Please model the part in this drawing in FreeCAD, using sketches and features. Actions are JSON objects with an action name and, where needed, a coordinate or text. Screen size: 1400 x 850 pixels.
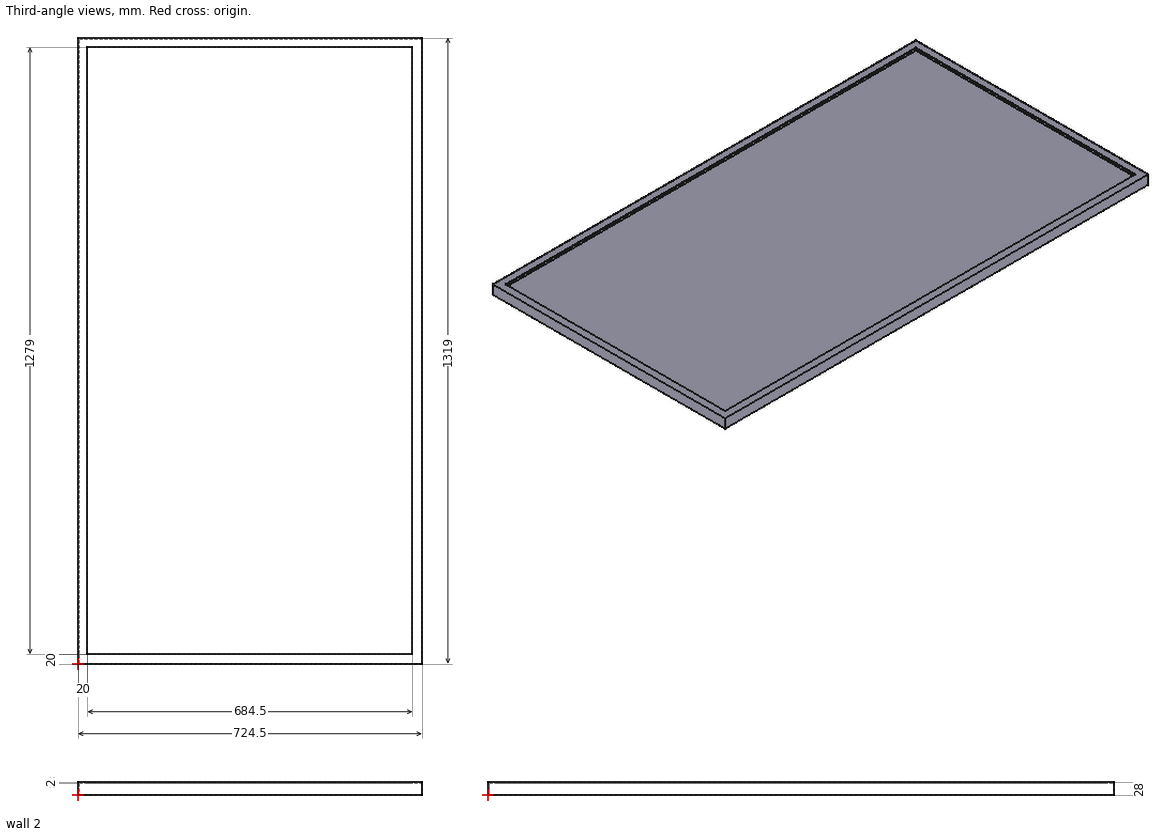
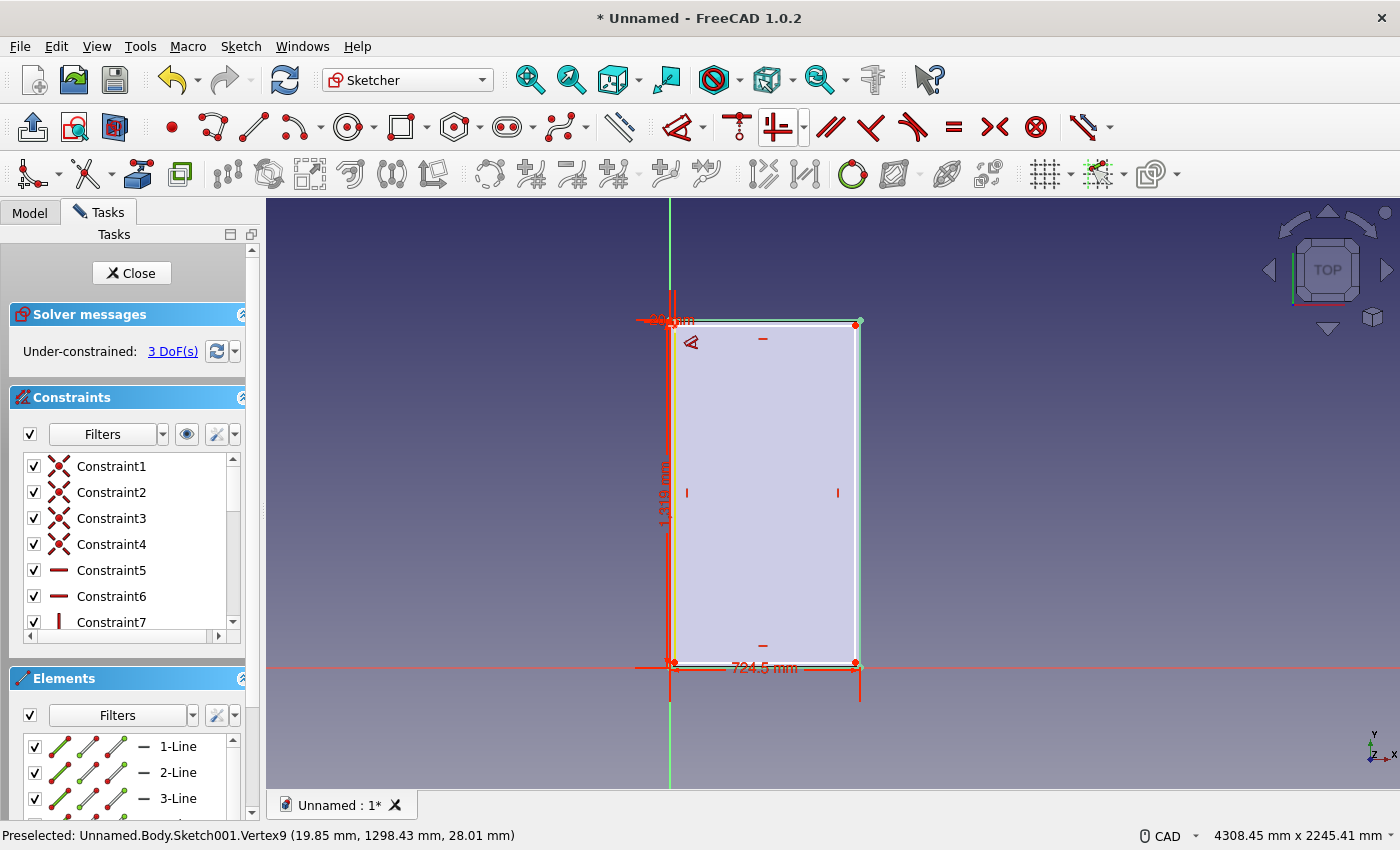
{"action": "scroll", "coordinate": [675, 663], "scroll_direction": "up", "scroll_amount": 11}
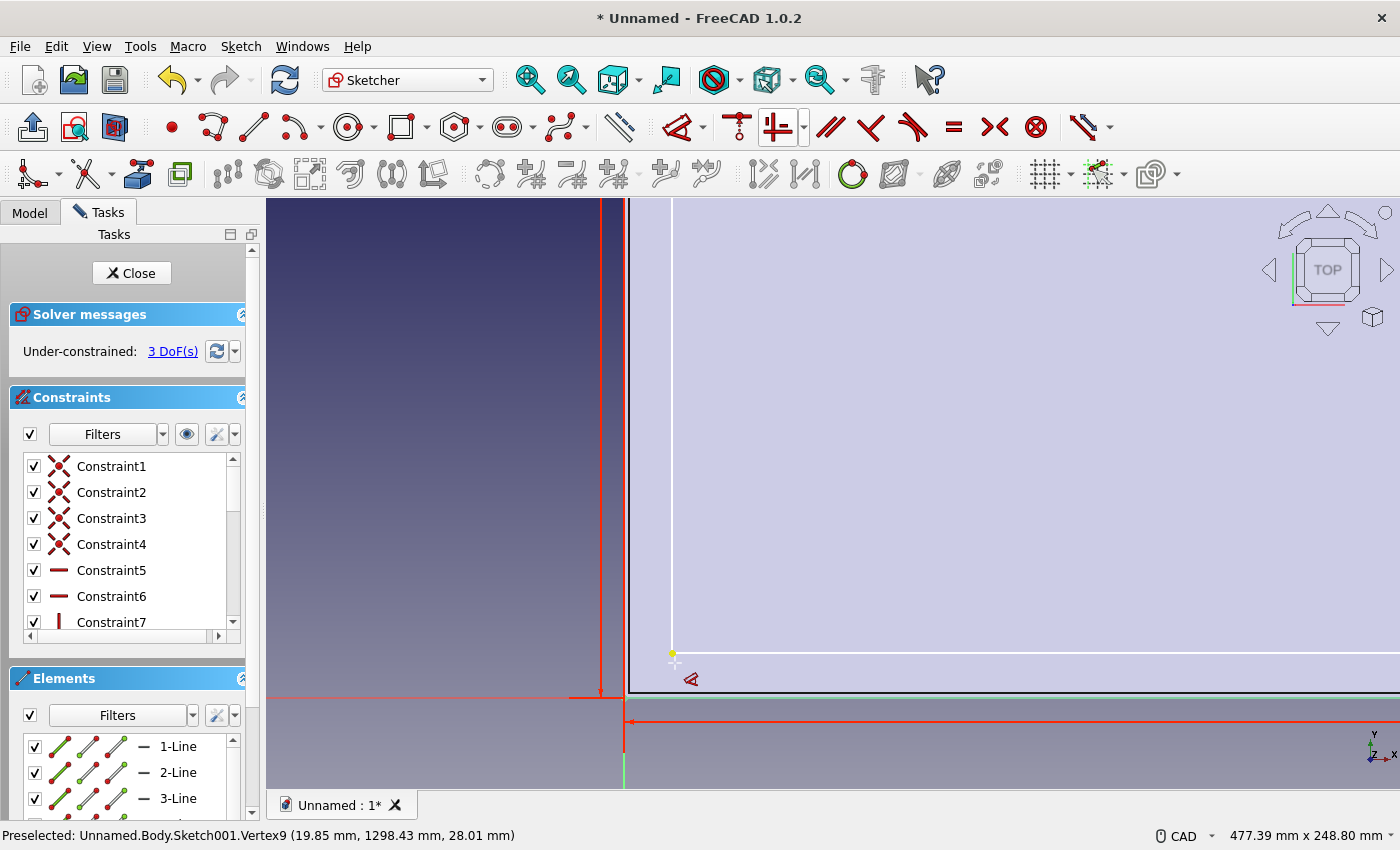
{"action": "left_click", "coordinate": [672, 653]}
{"action": "left_click", "coordinate": [590, 676]}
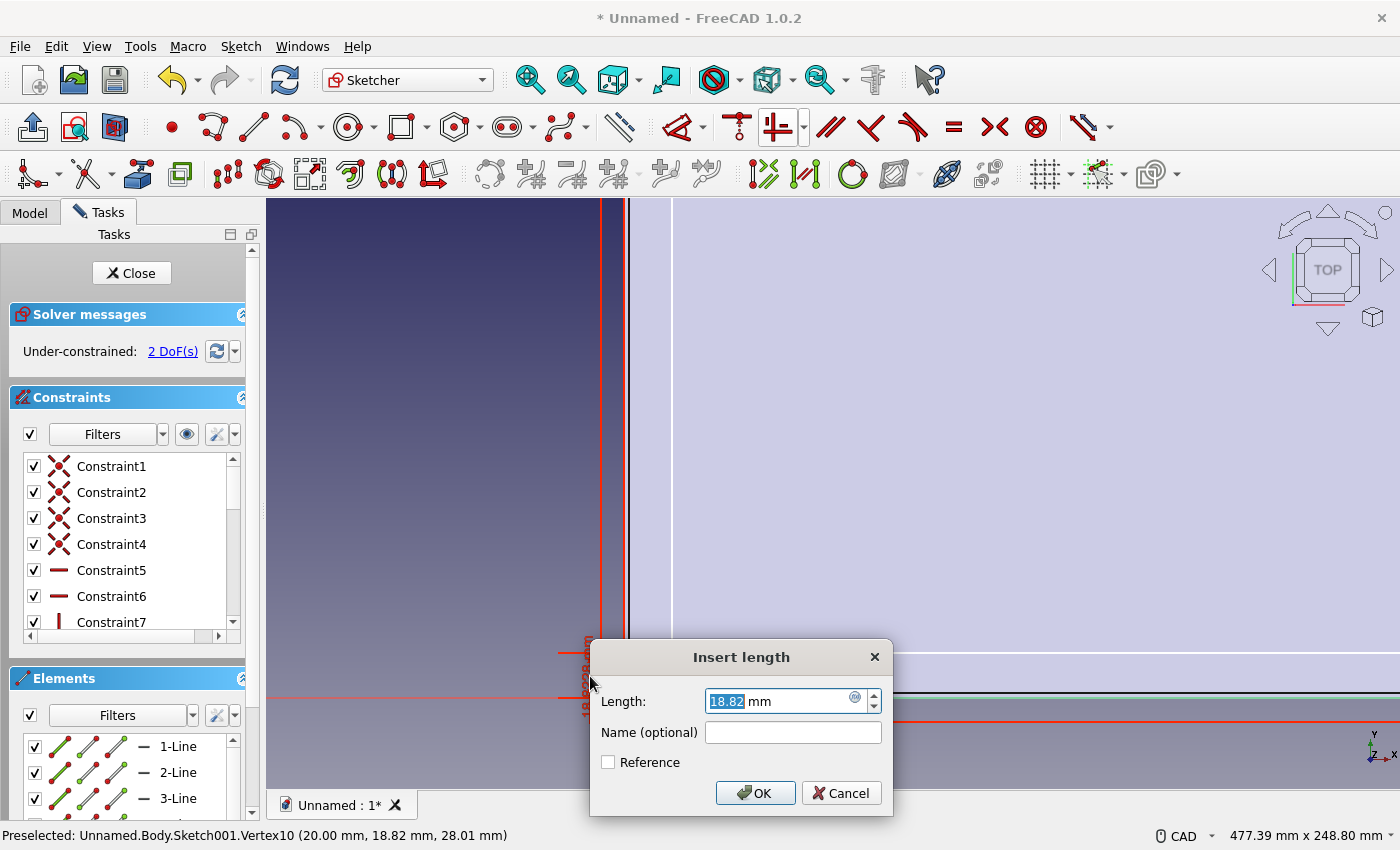
{"action": "type", "text": "20"}
{"action": "key", "text": "Return"}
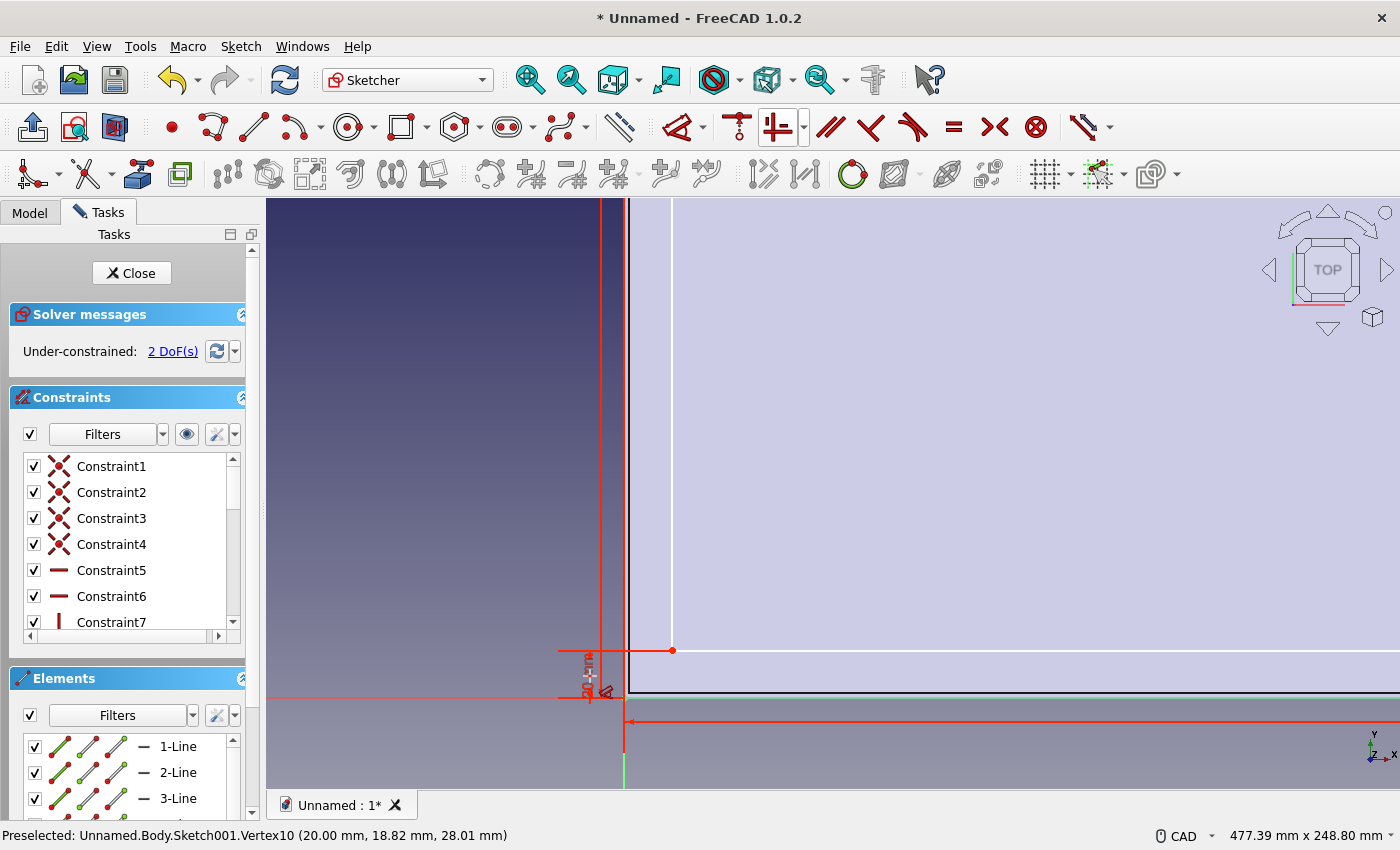
{"action": "scroll", "coordinate": [675, 663], "scroll_direction": "down", "scroll_amount": 11}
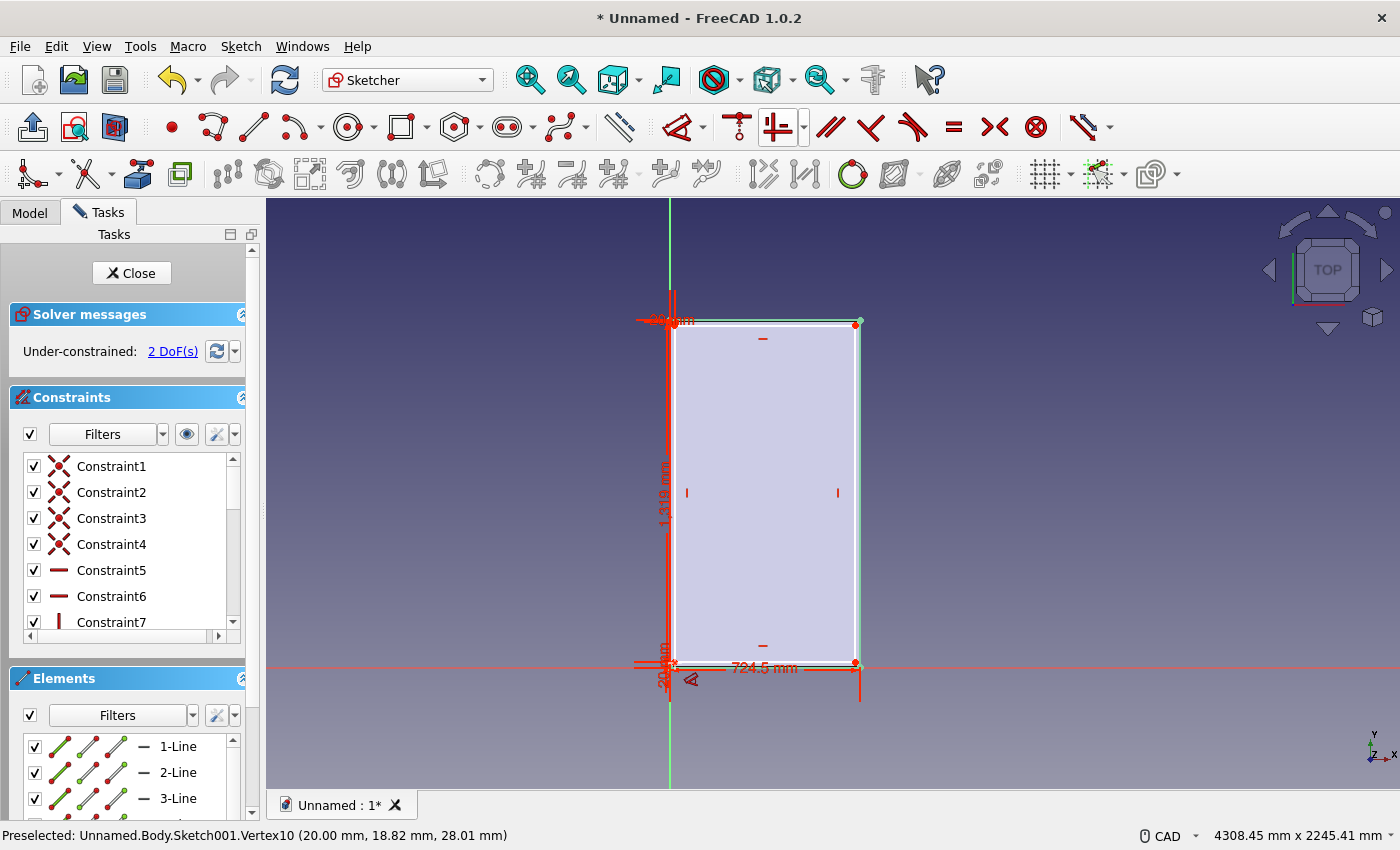
{"action": "scroll", "coordinate": [675, 427], "scroll_direction": "up", "scroll_amount": 5}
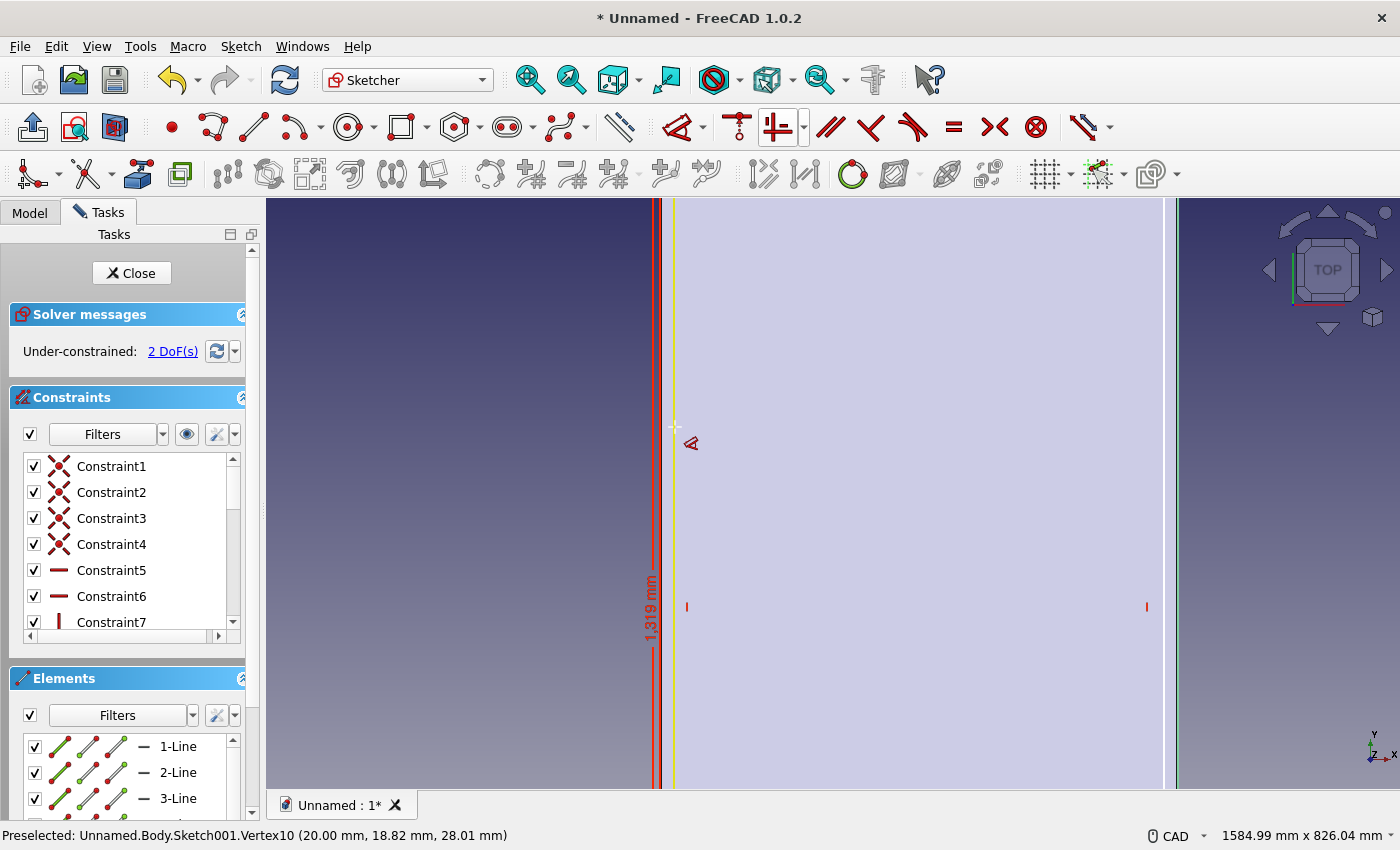
{"action": "left_click", "coordinate": [674, 426]}
{"action": "left_click", "coordinate": [640, 494]}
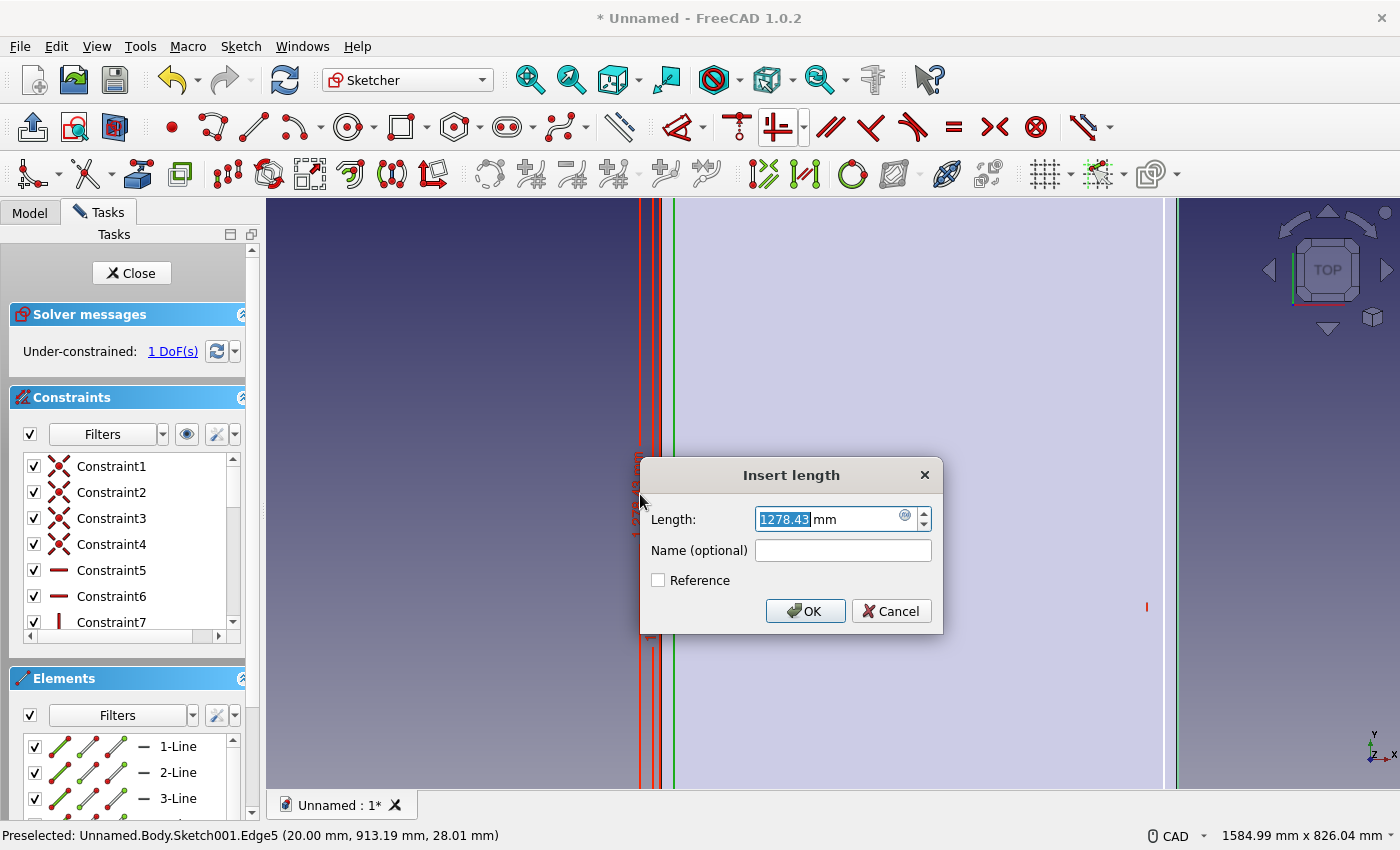
{"action": "type", "text": "1279"}
{"action": "key", "text": "Return"}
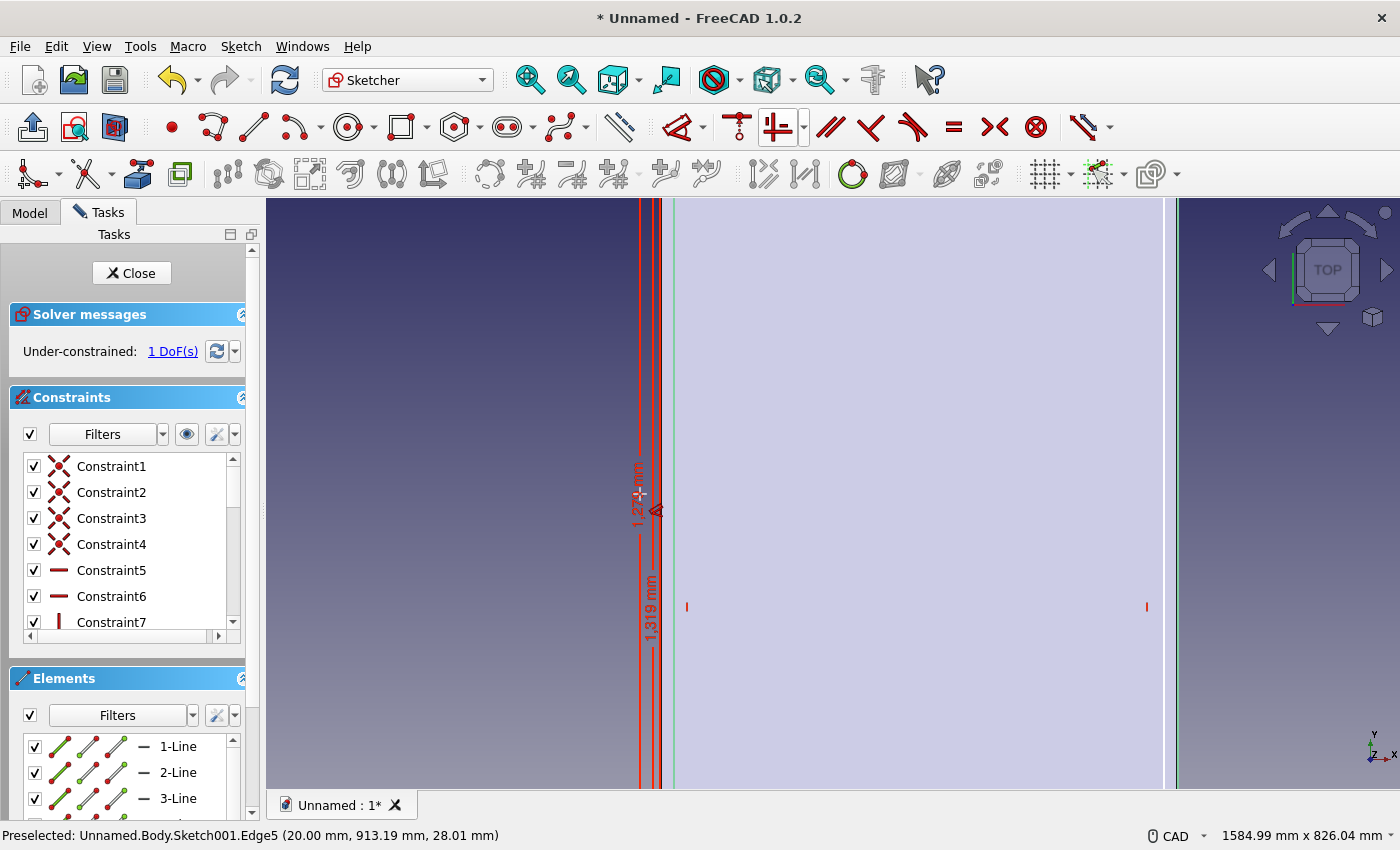
{"action": "scroll", "coordinate": [674, 427], "scroll_direction": "down", "scroll_amount": 5}